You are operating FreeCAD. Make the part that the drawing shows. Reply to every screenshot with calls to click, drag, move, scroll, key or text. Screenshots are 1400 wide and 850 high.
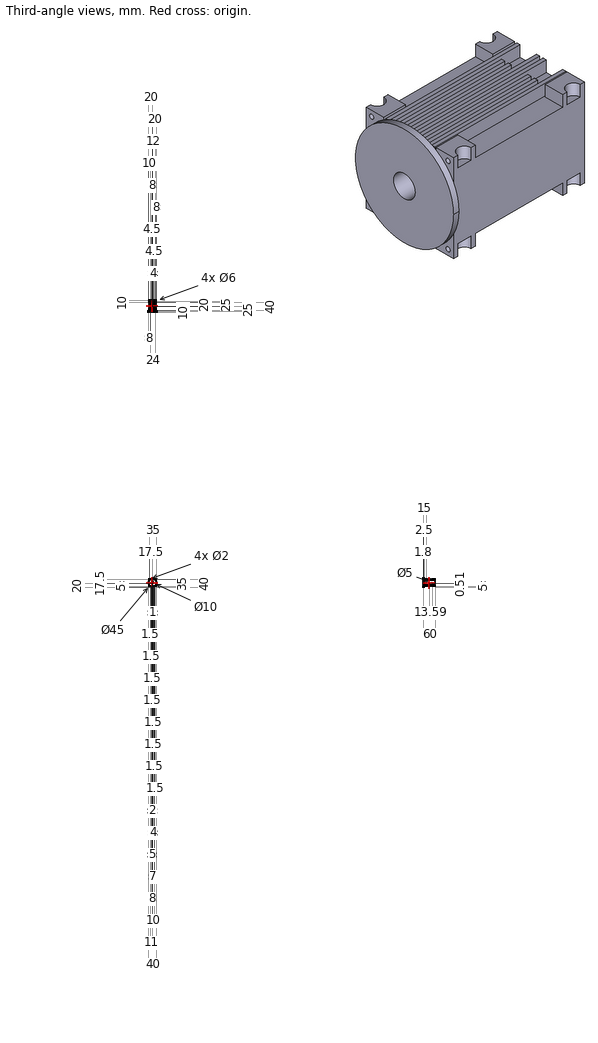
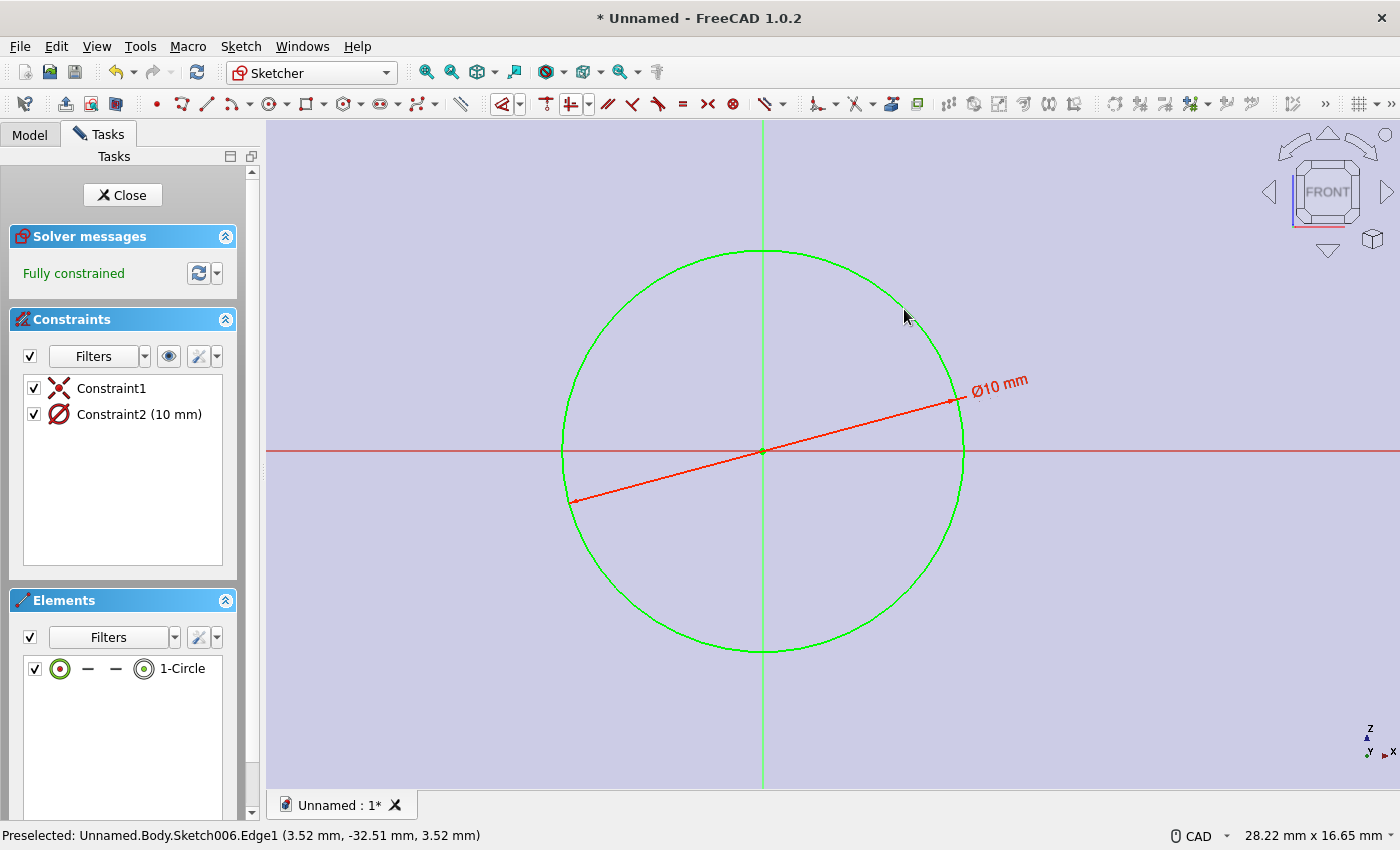
click(123, 195)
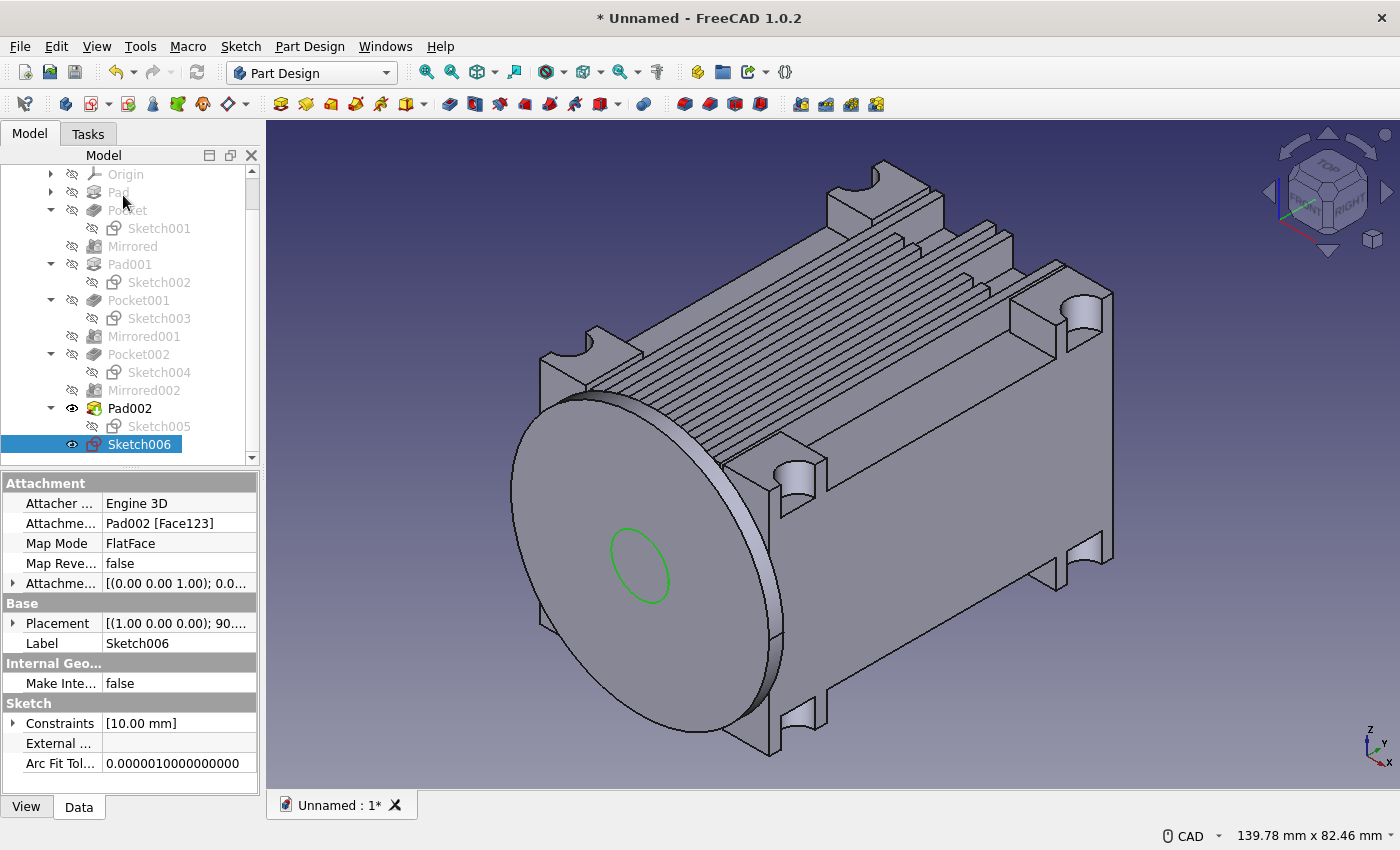
click(450, 104)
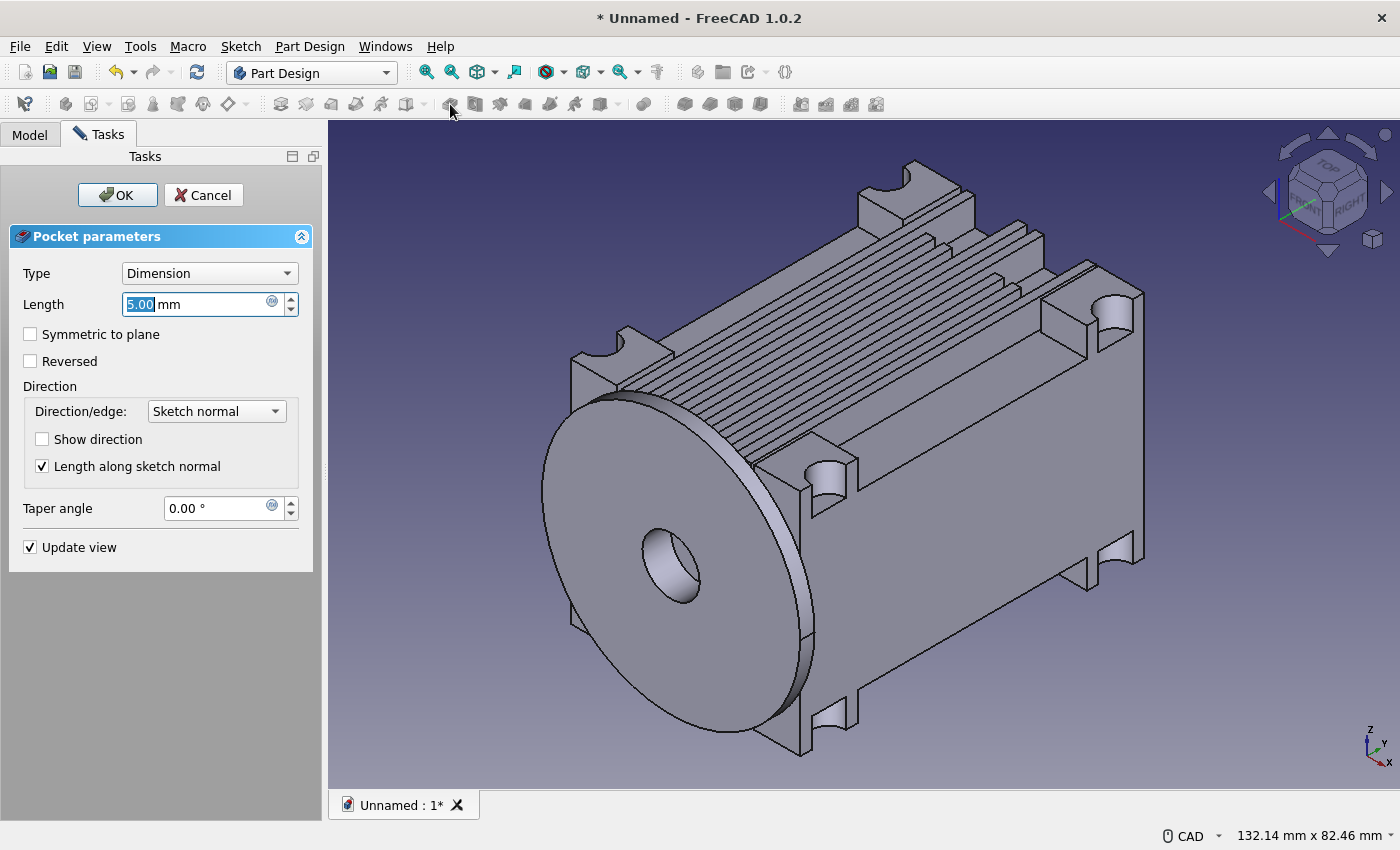
text(15)
key(Tab)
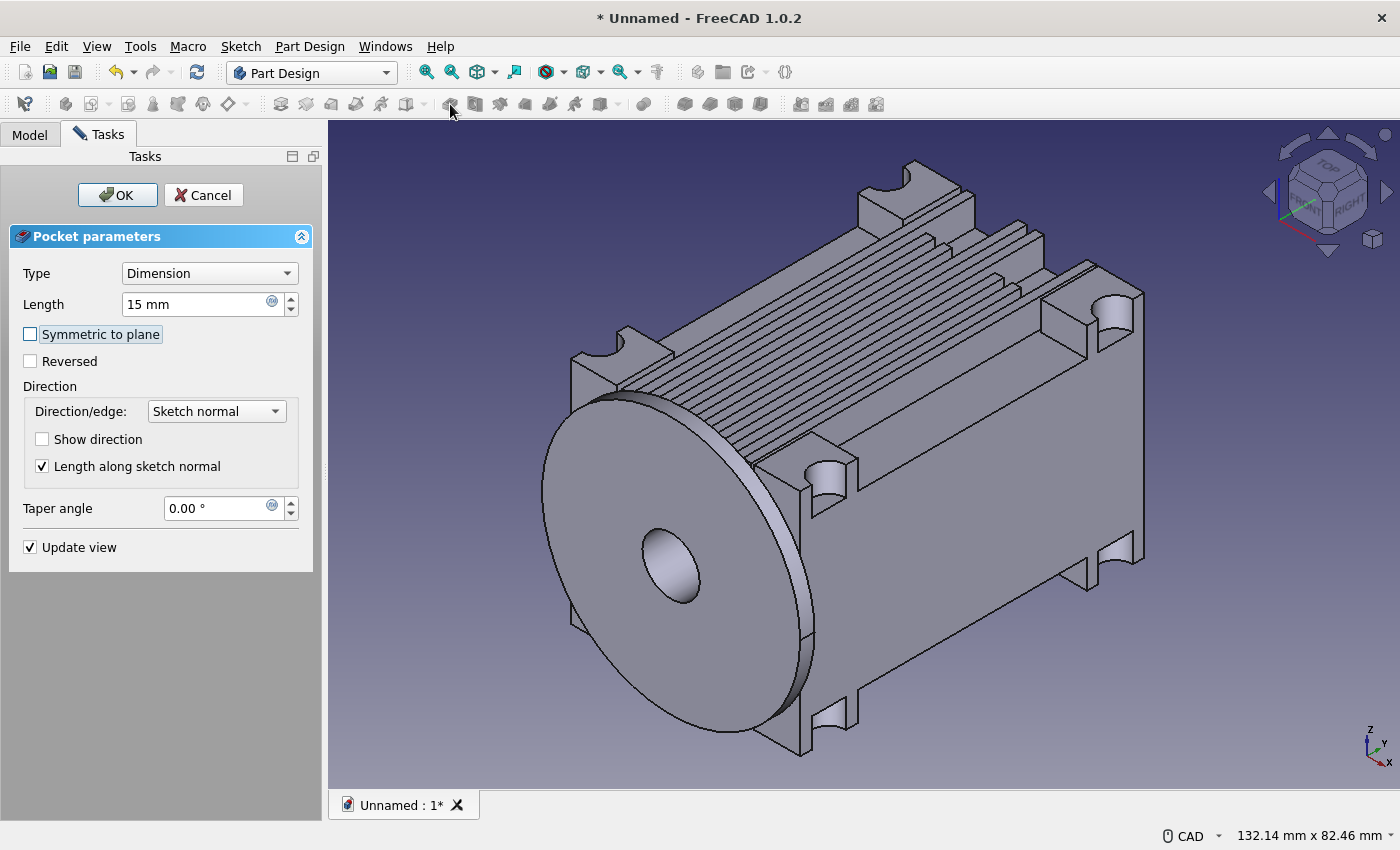
click(118, 195)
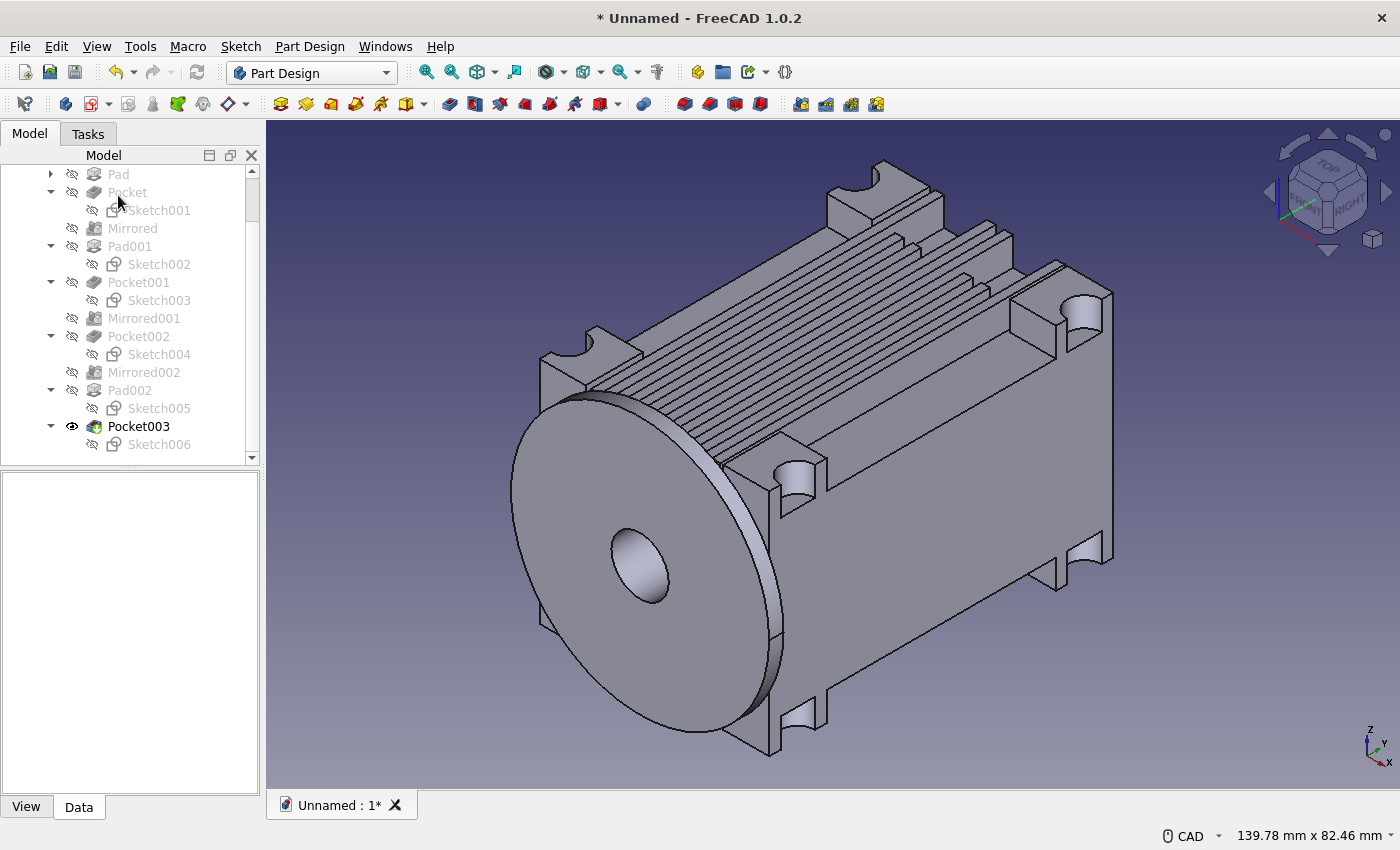
key(6)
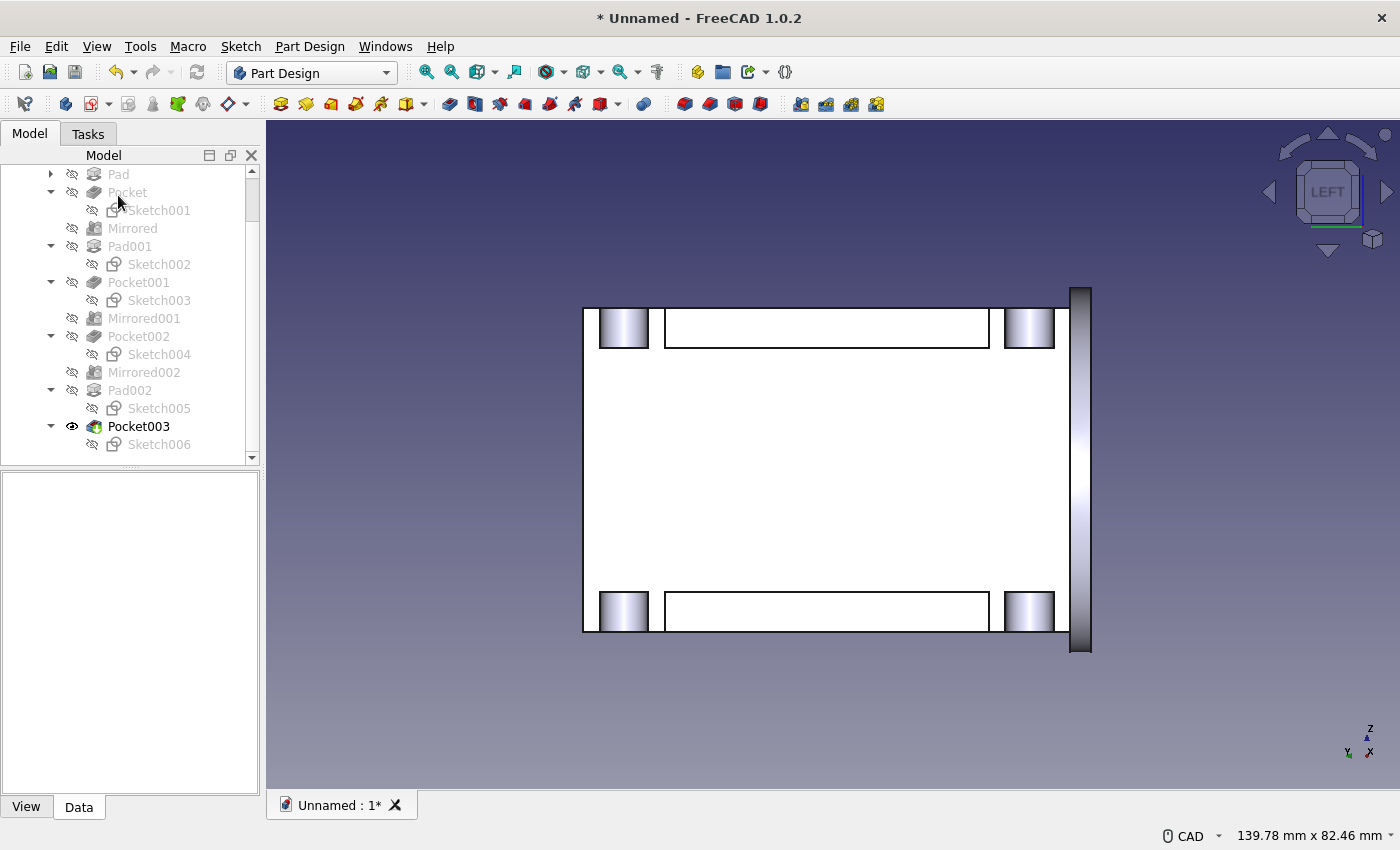
click(896, 469)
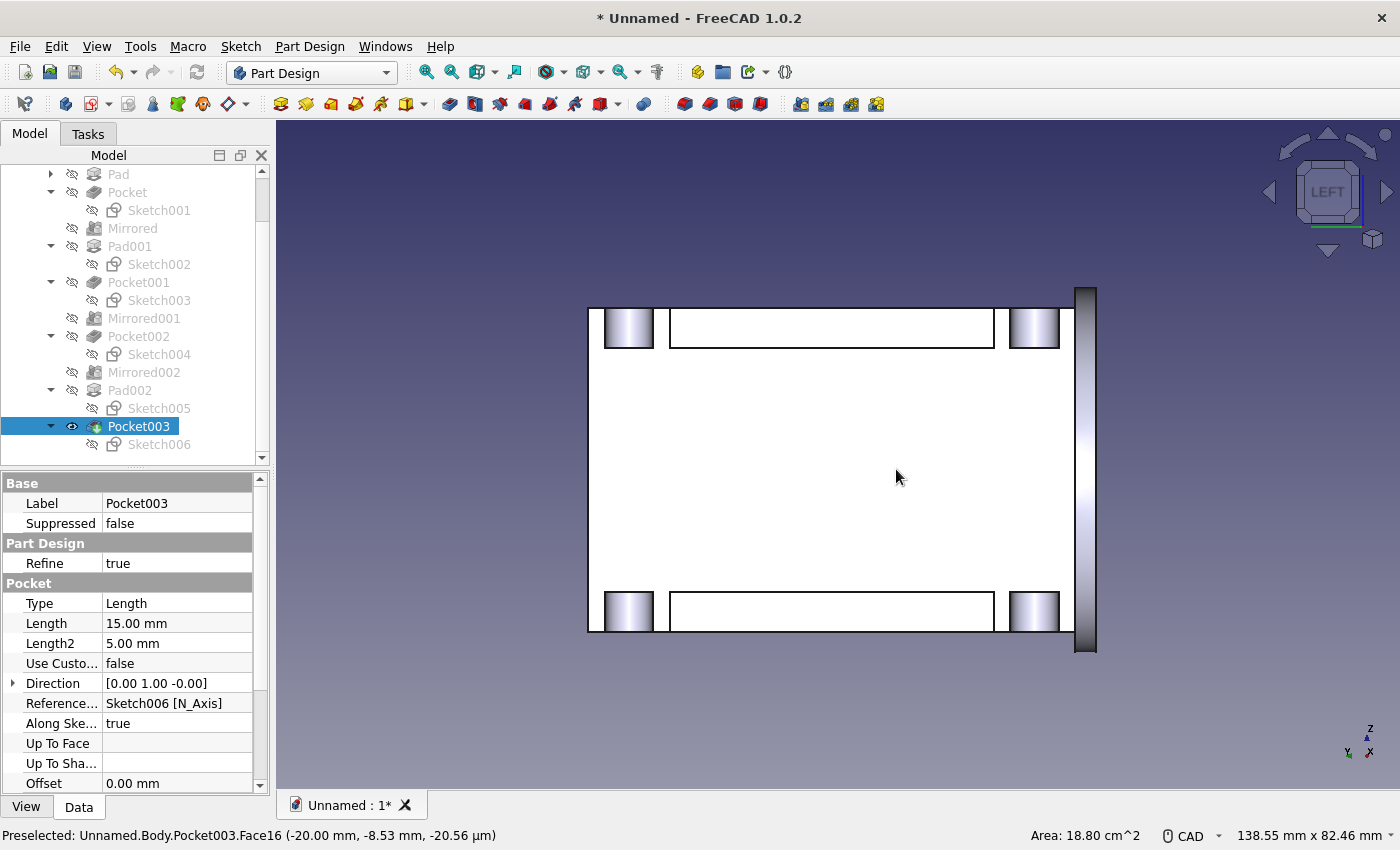
click(90, 104)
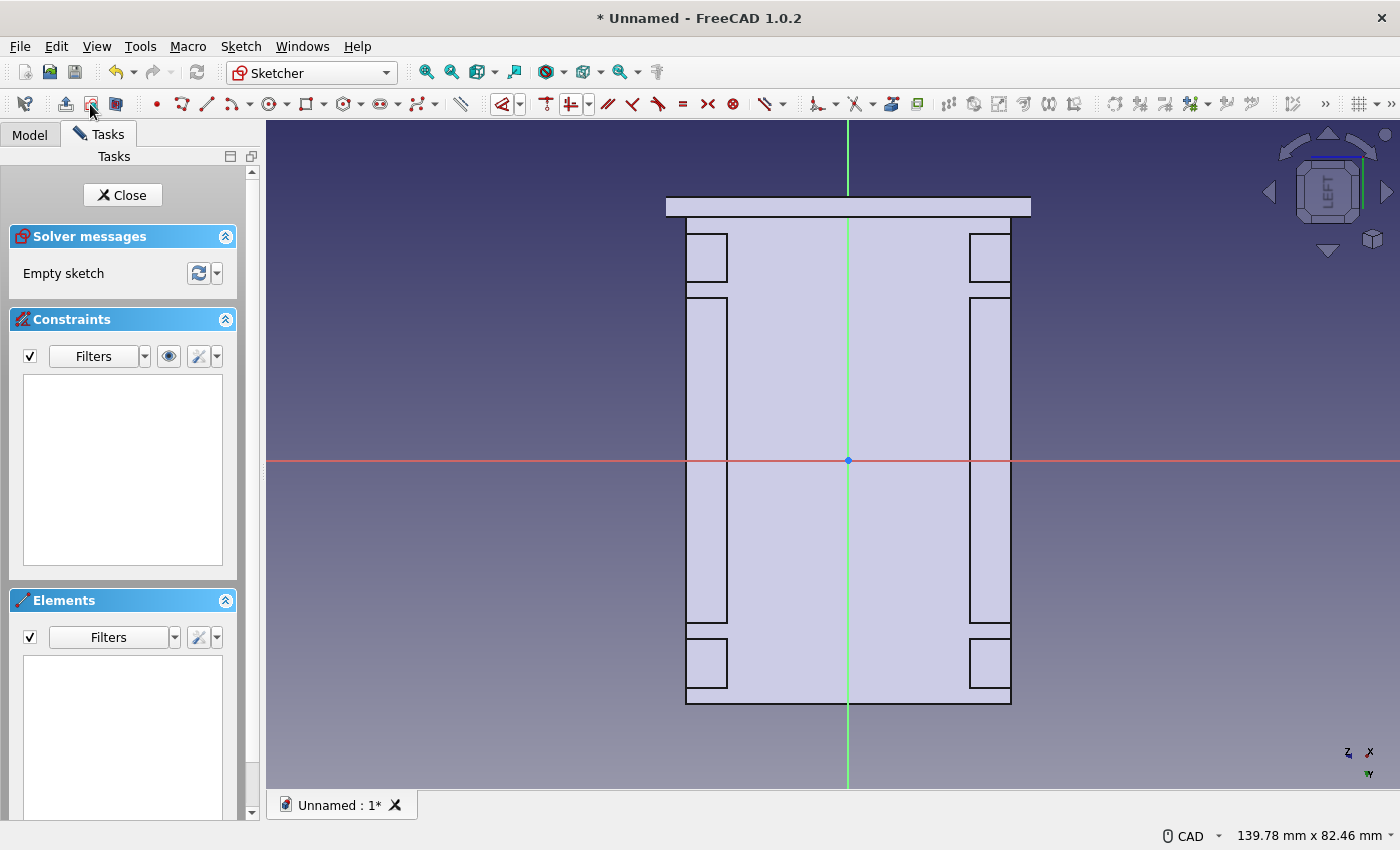
key(q)
key(s)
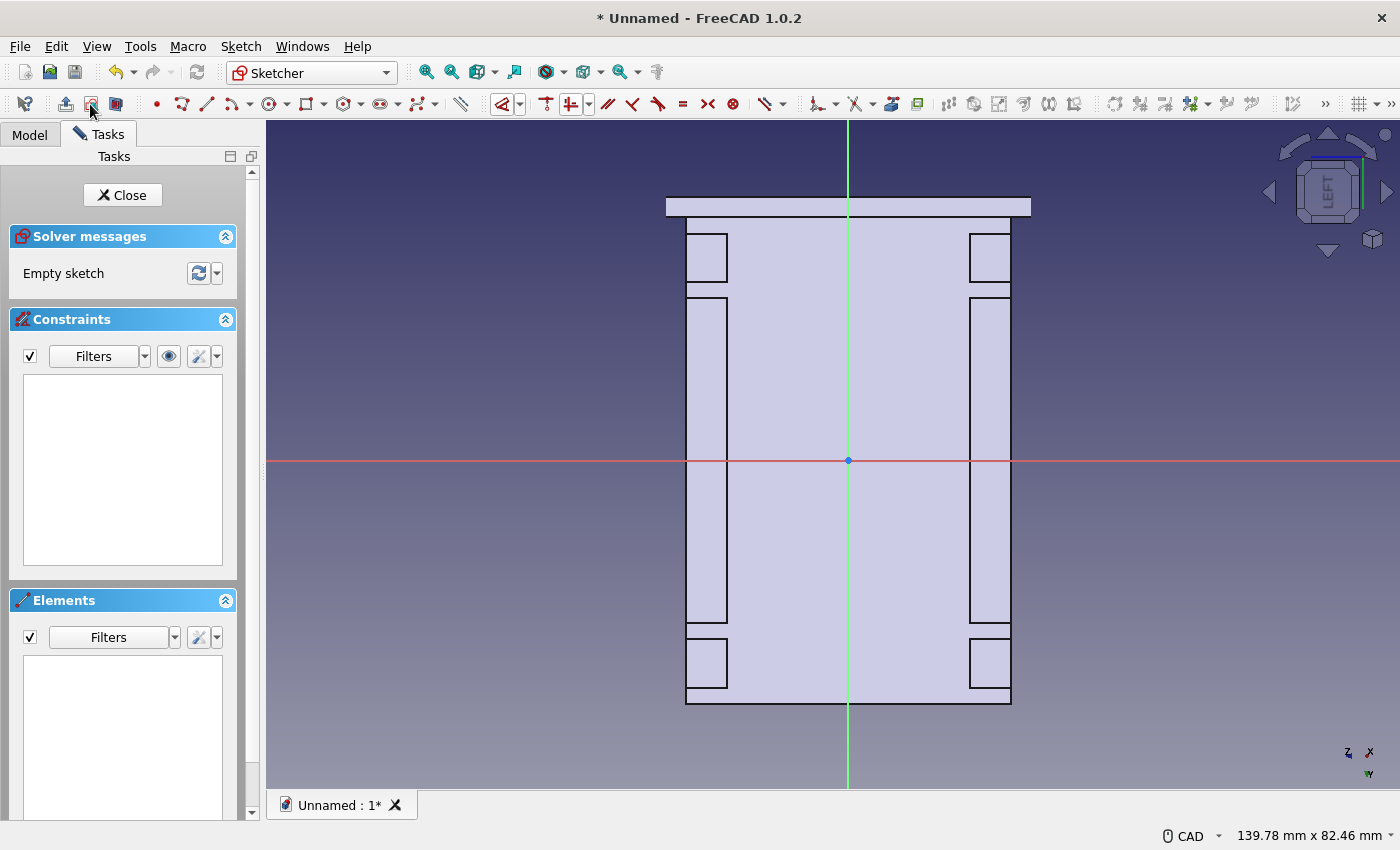
scroll(861, 583, up, 12)